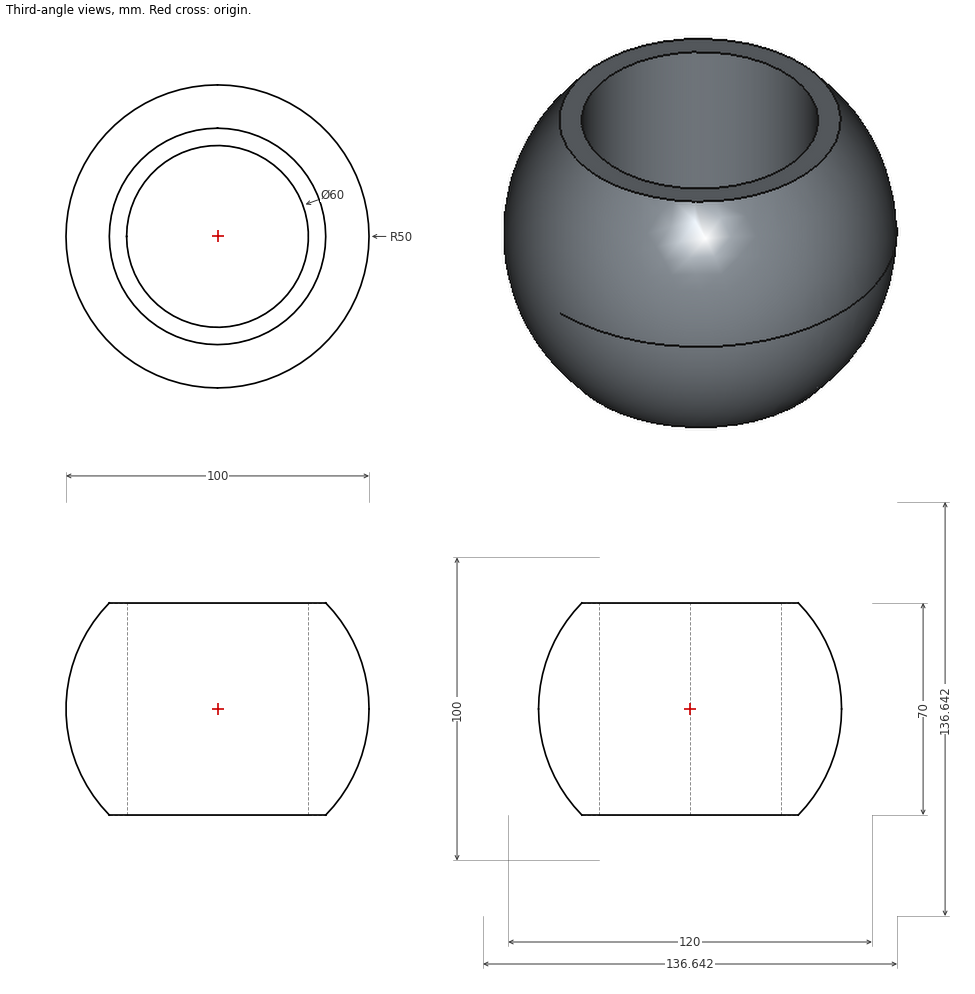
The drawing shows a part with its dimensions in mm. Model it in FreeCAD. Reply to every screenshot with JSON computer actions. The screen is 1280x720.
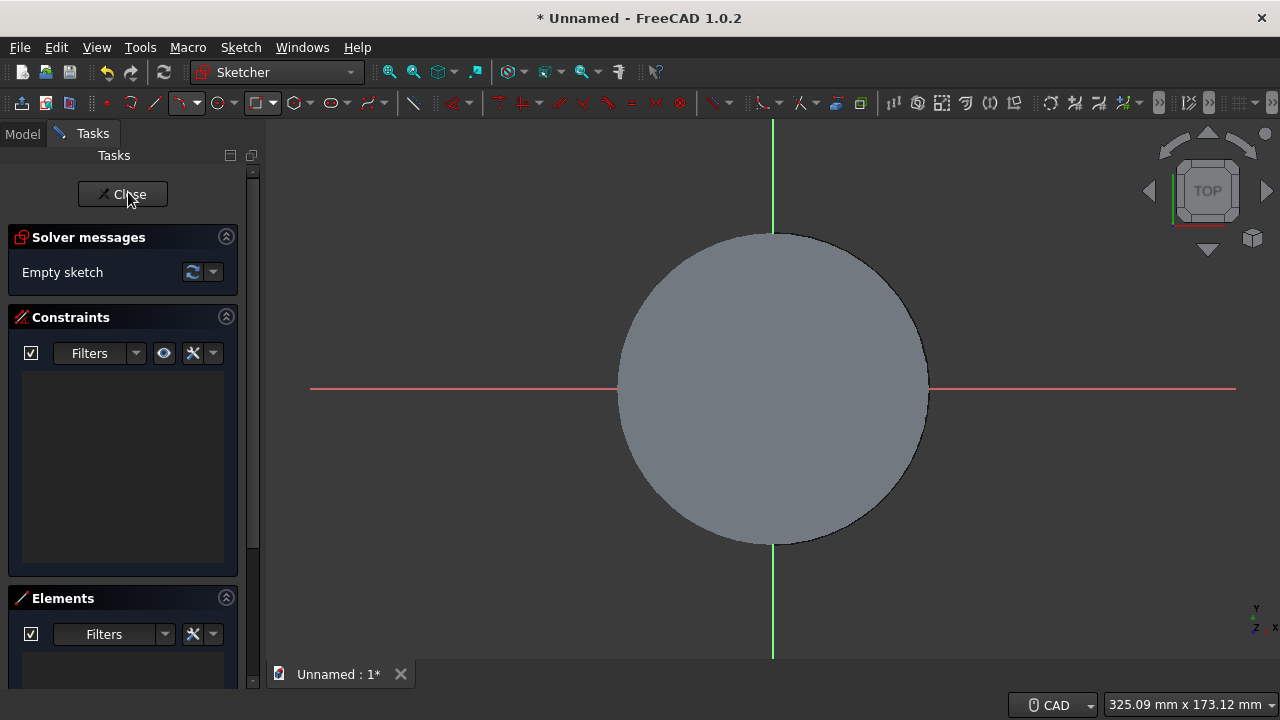
{"action": "left_click", "coordinate": [70, 104]}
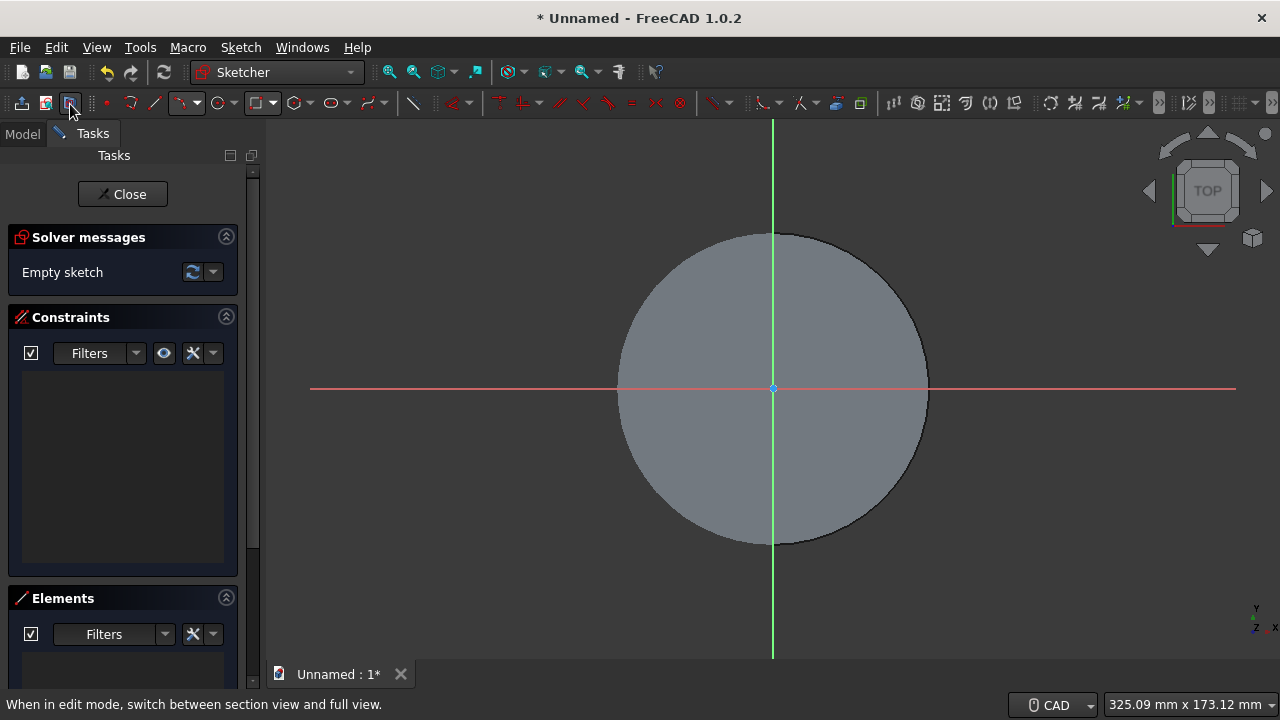
{"action": "scroll", "coordinate": [857, 389], "scroll_direction": "up", "scroll_amount": 3}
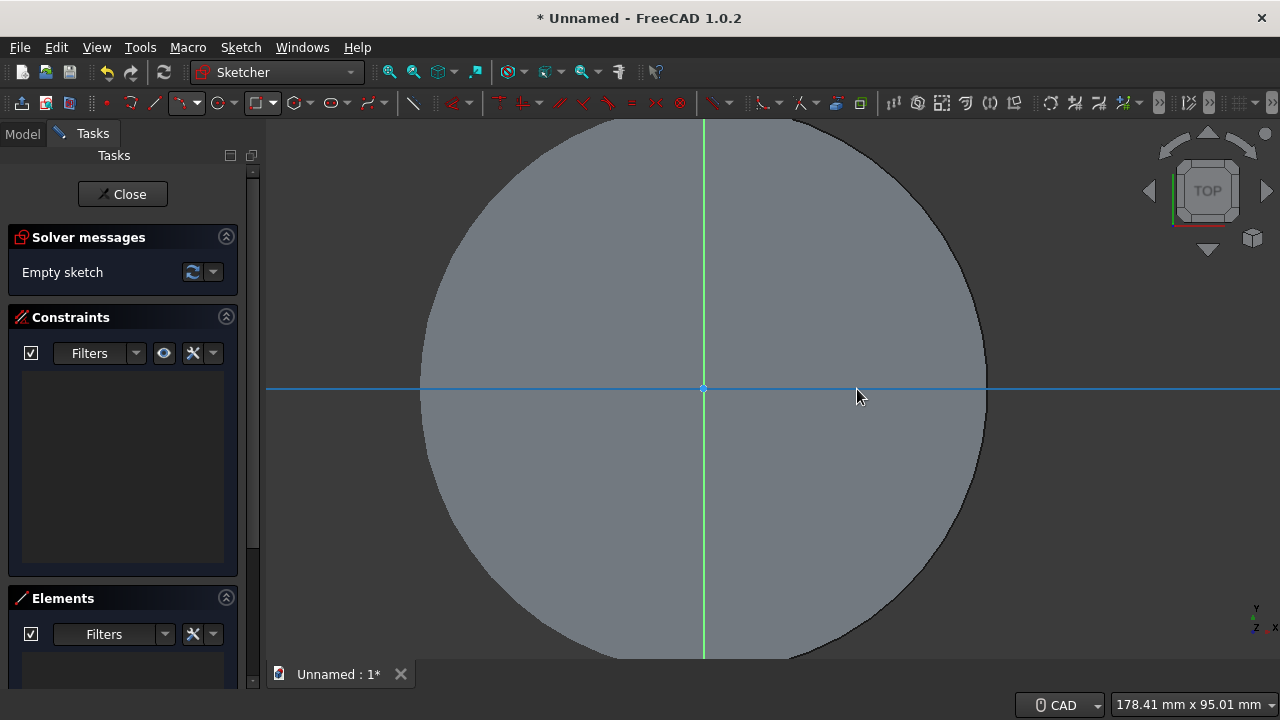
{"action": "left_click", "coordinate": [218, 104]}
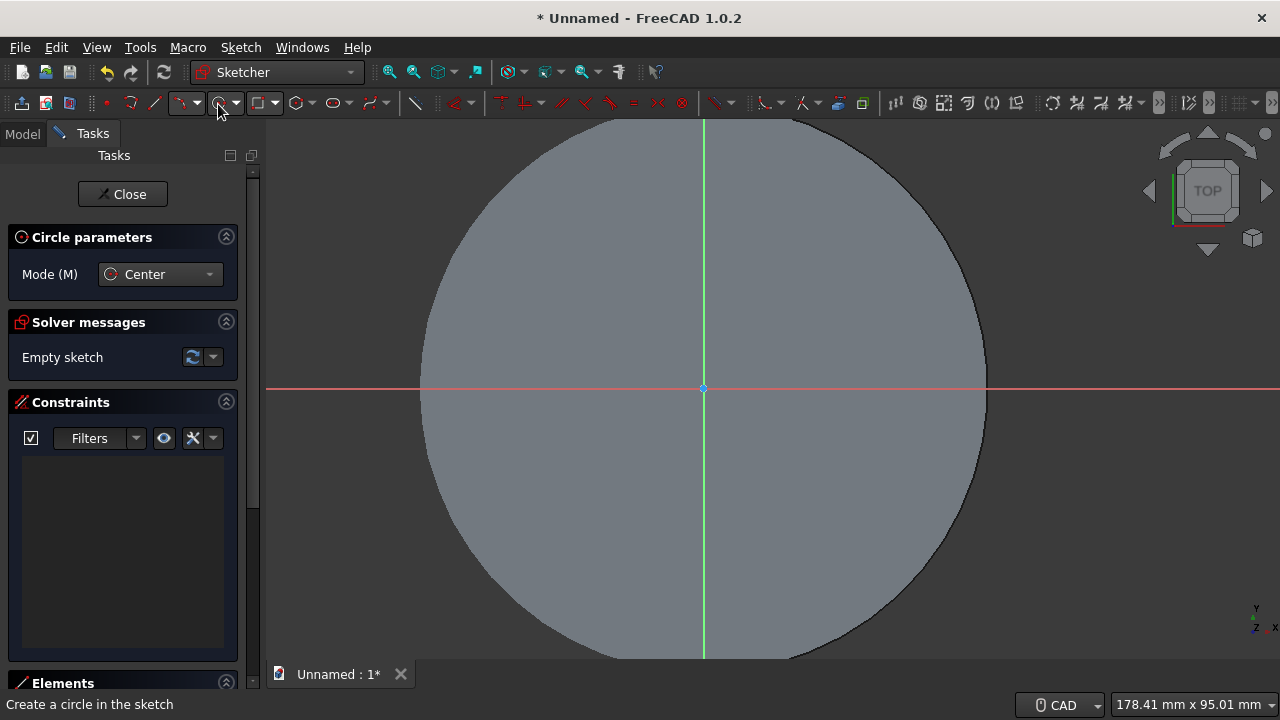
{"action": "left_click", "coordinate": [704, 389]}
{"action": "left_click", "coordinate": [824, 268]}
{"action": "key", "text": "Escape"}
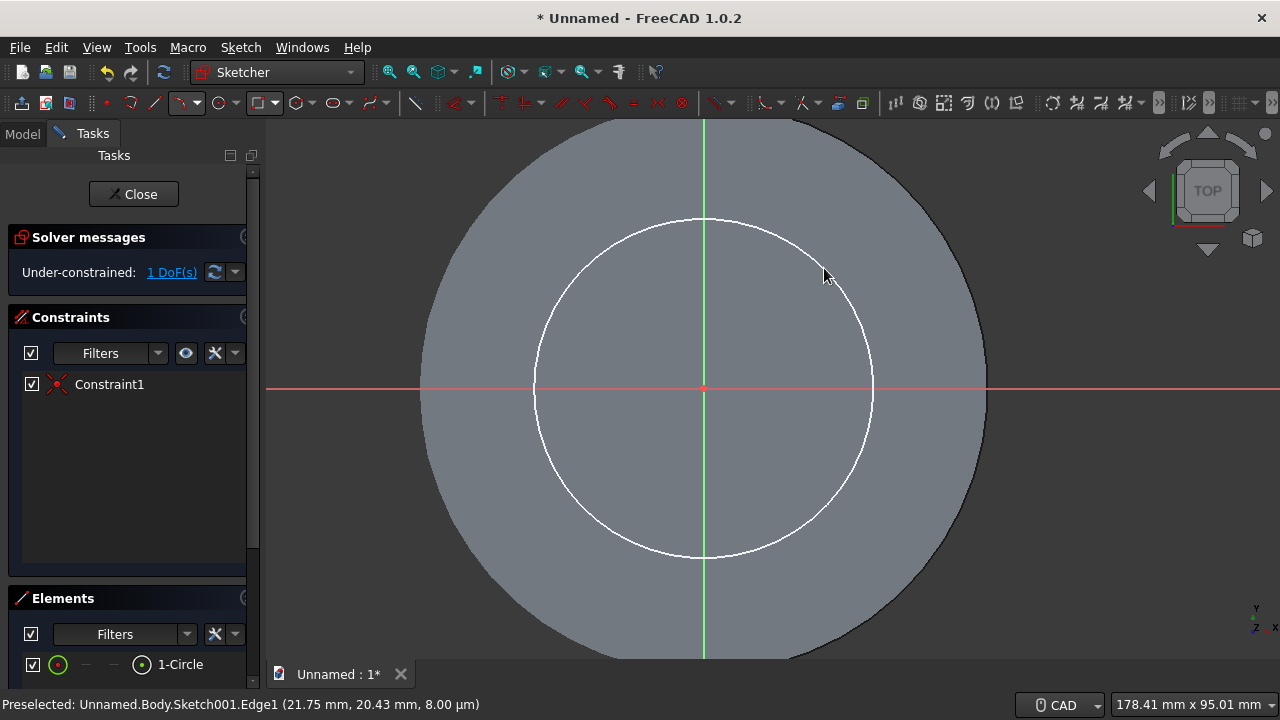
{"action": "left_click", "coordinate": [454, 104]}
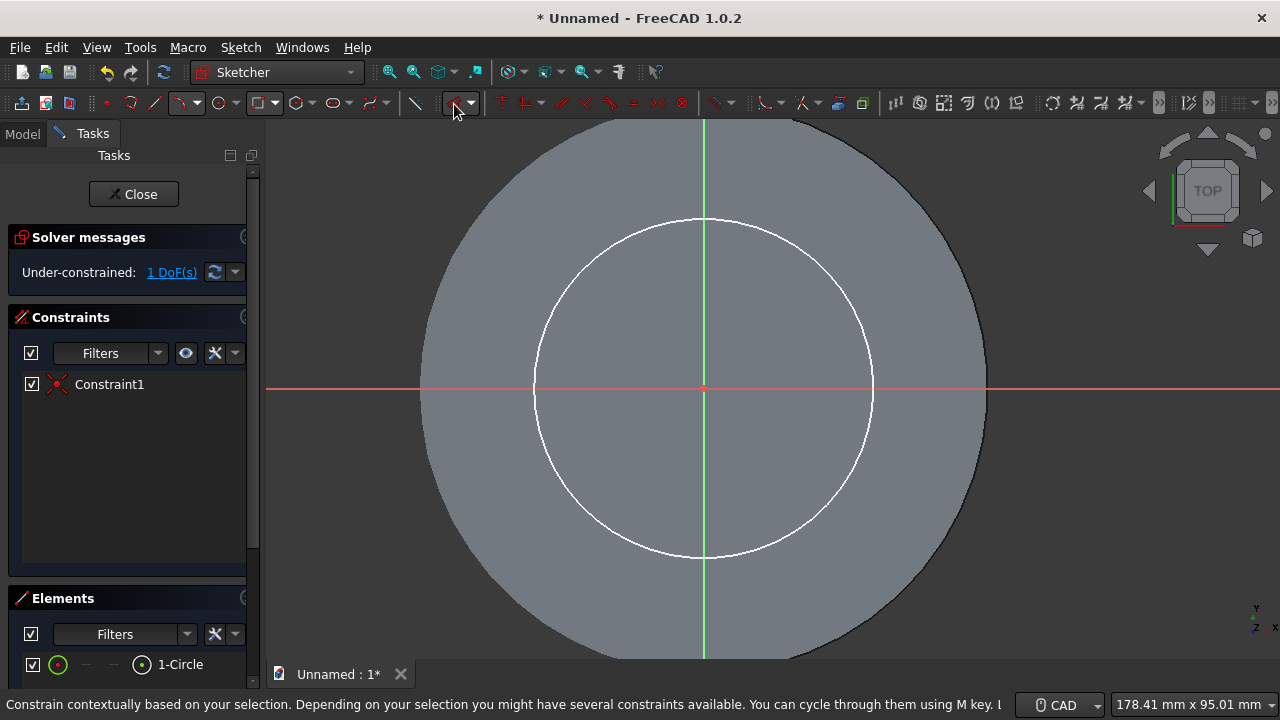
{"action": "left_click", "coordinate": [823, 268]}
{"action": "left_click", "coordinate": [846, 245]}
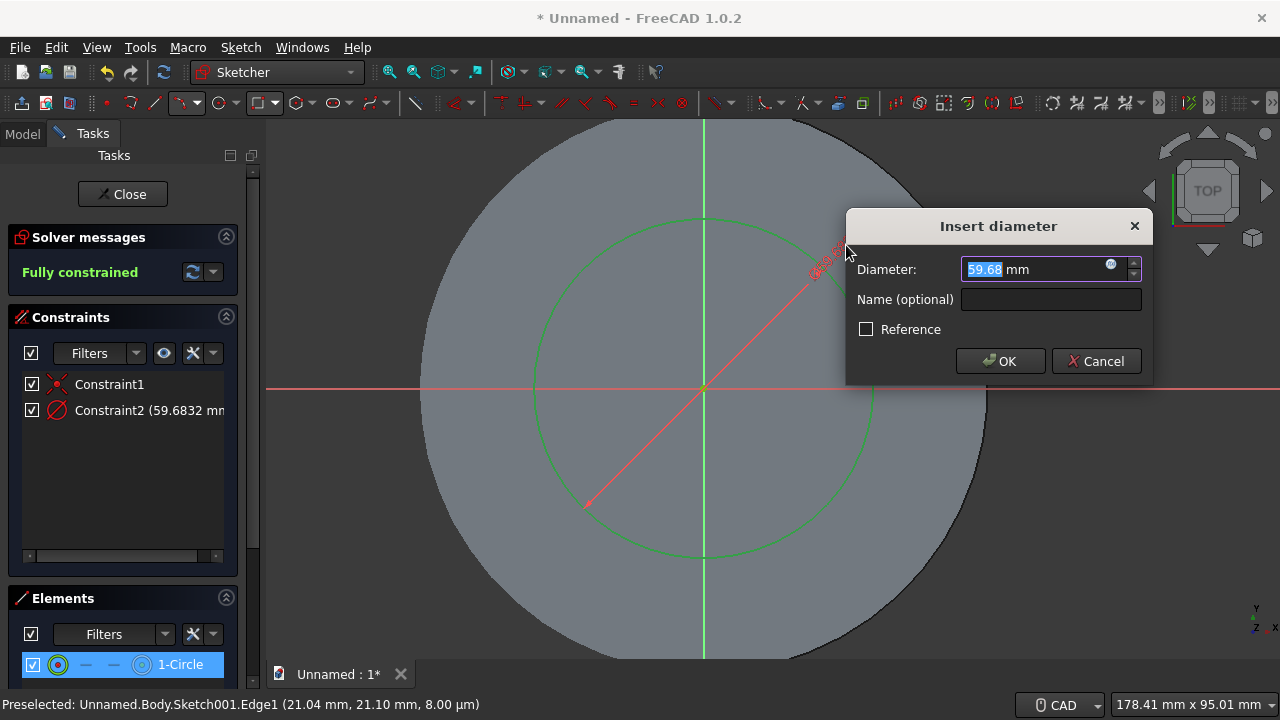
{"action": "type", "text": "60"}
{"action": "key", "text": "Return"}
{"action": "key", "text": "Escape"}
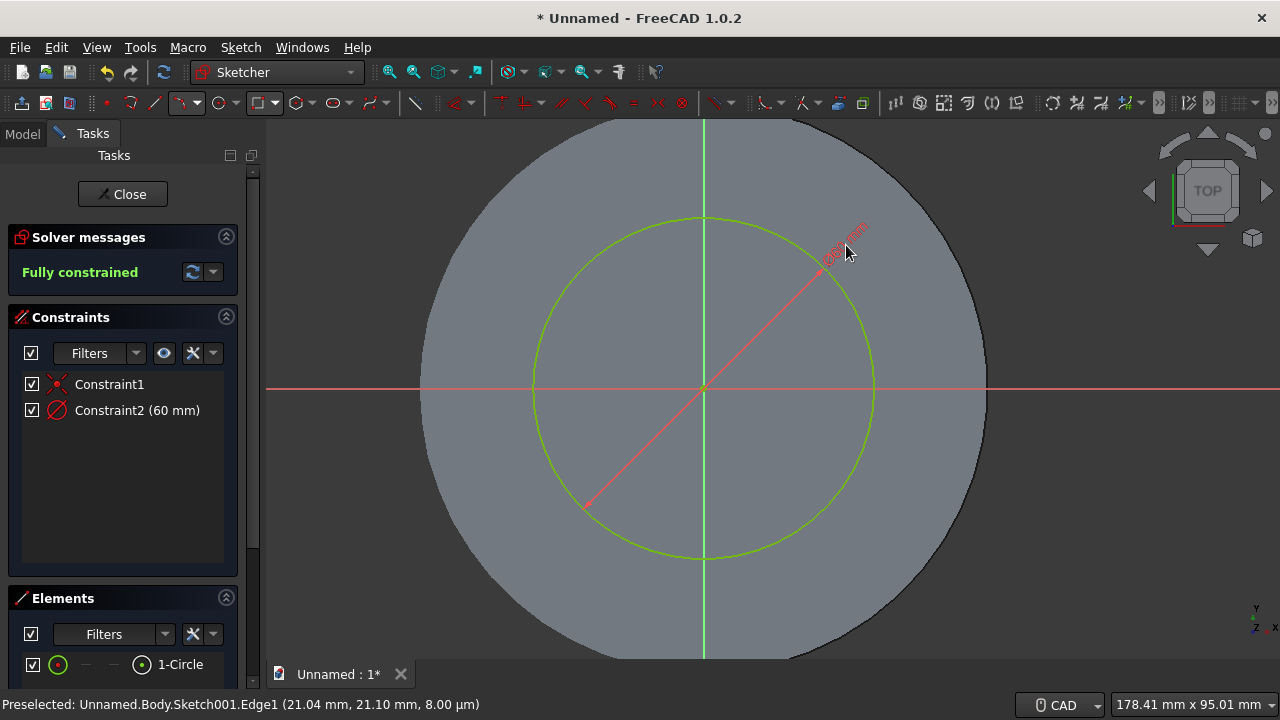
{"action": "left_click", "coordinate": [123, 194]}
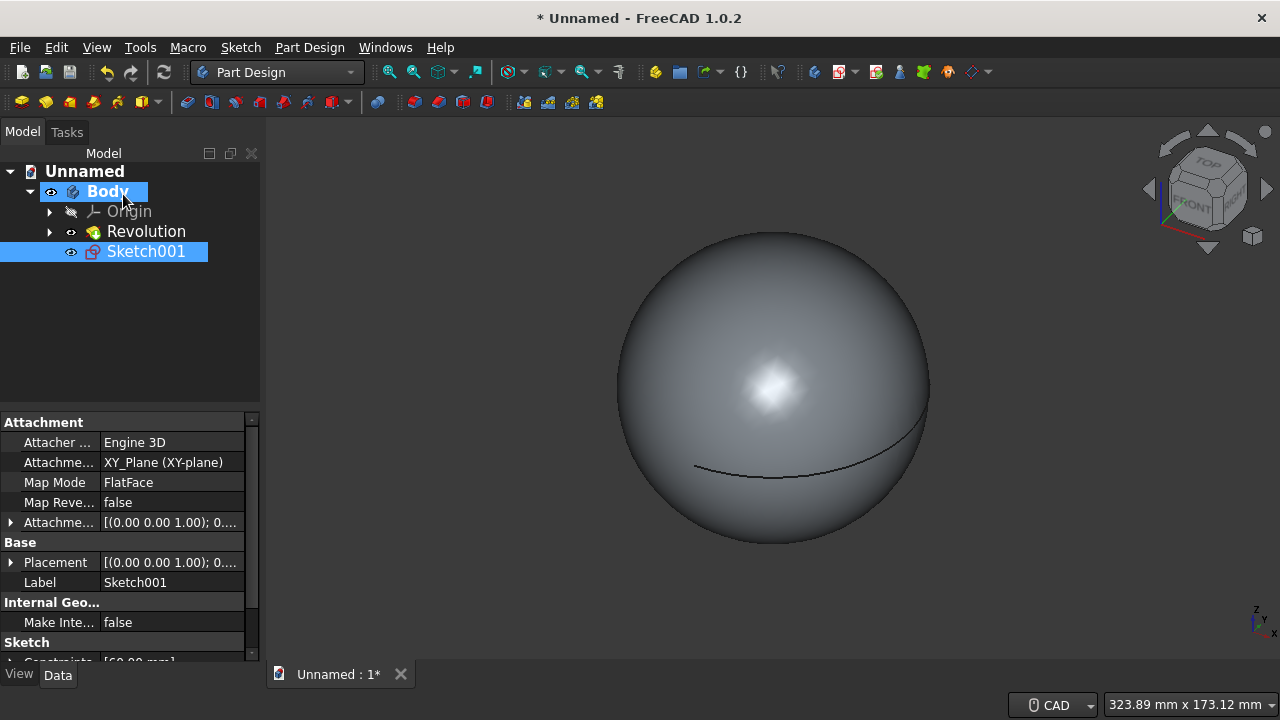
{"action": "left_click", "coordinate": [188, 102]}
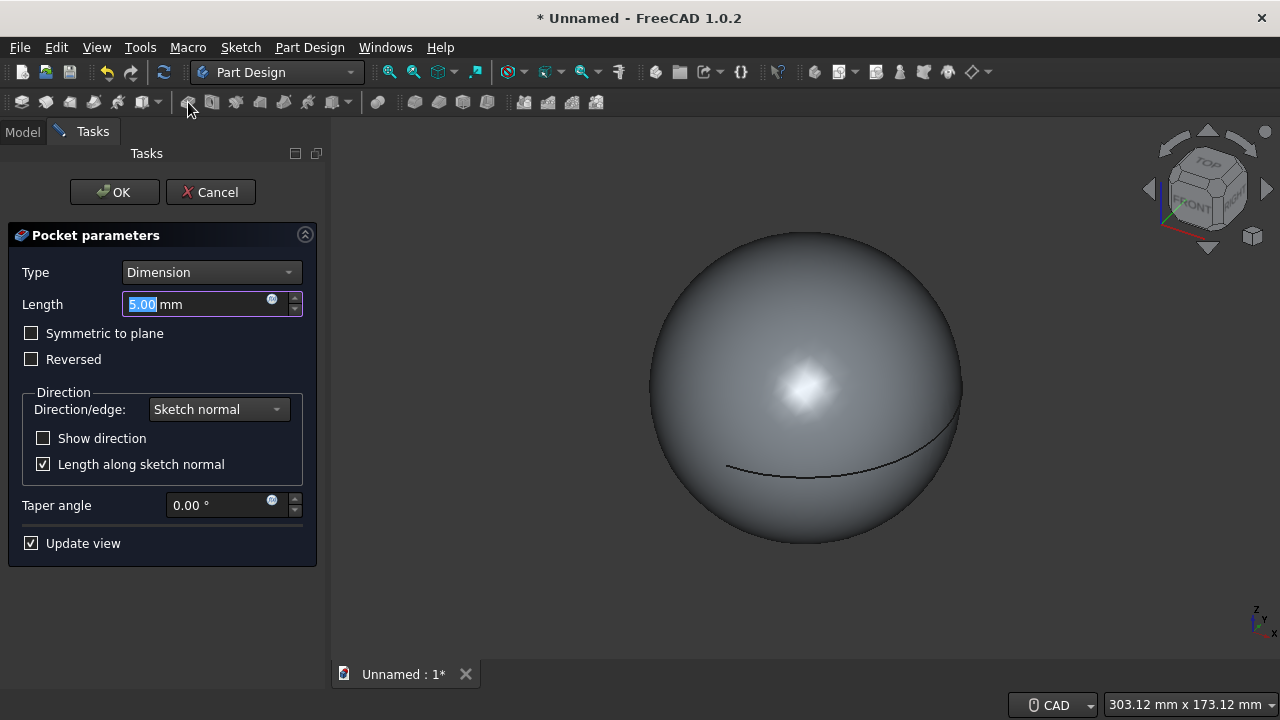
{"action": "type", "text": "100"}
{"action": "key", "text": "Tab"}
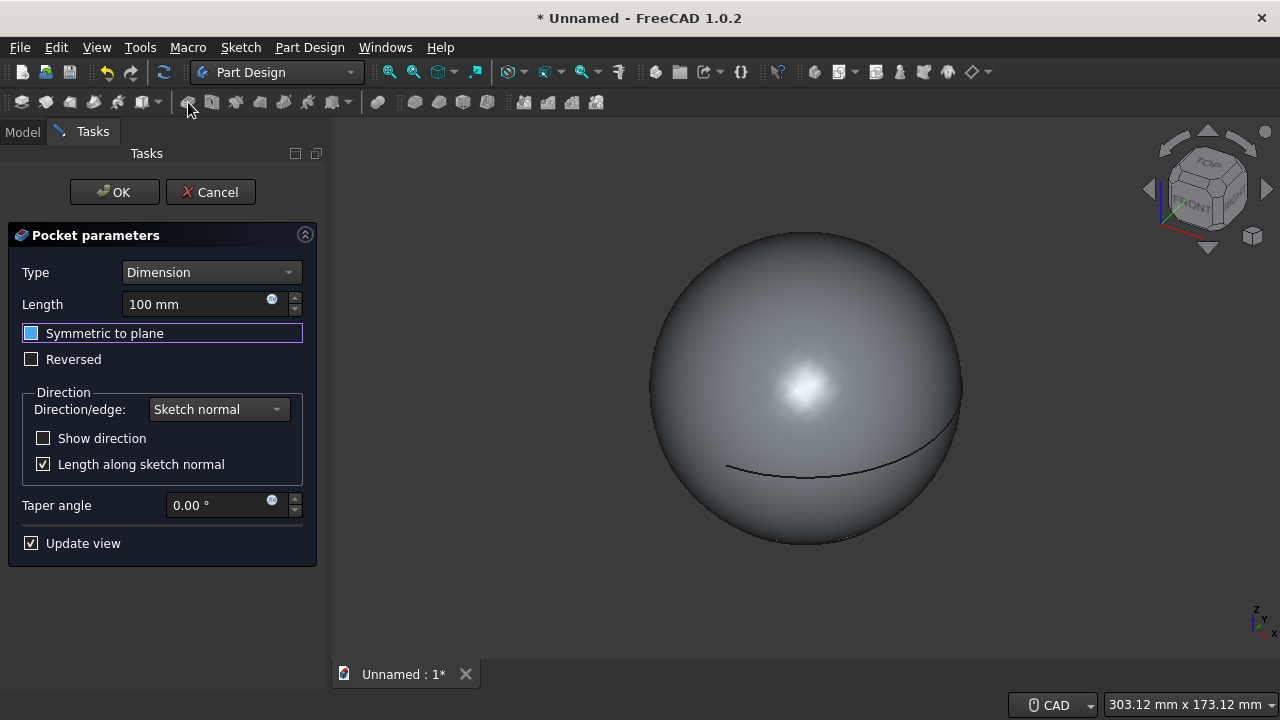
{"action": "left_click", "coordinate": [30, 333]}